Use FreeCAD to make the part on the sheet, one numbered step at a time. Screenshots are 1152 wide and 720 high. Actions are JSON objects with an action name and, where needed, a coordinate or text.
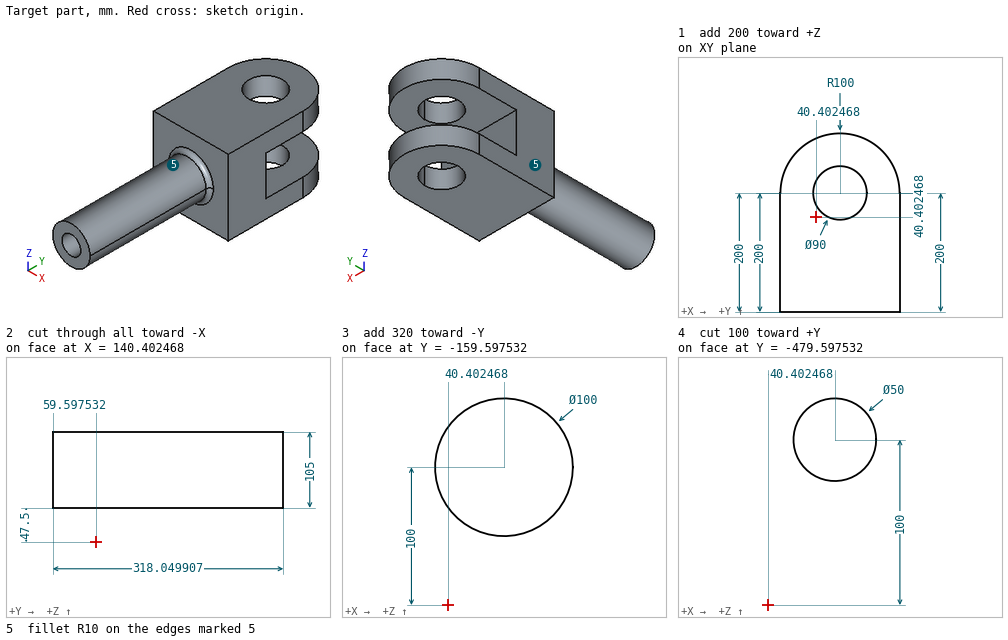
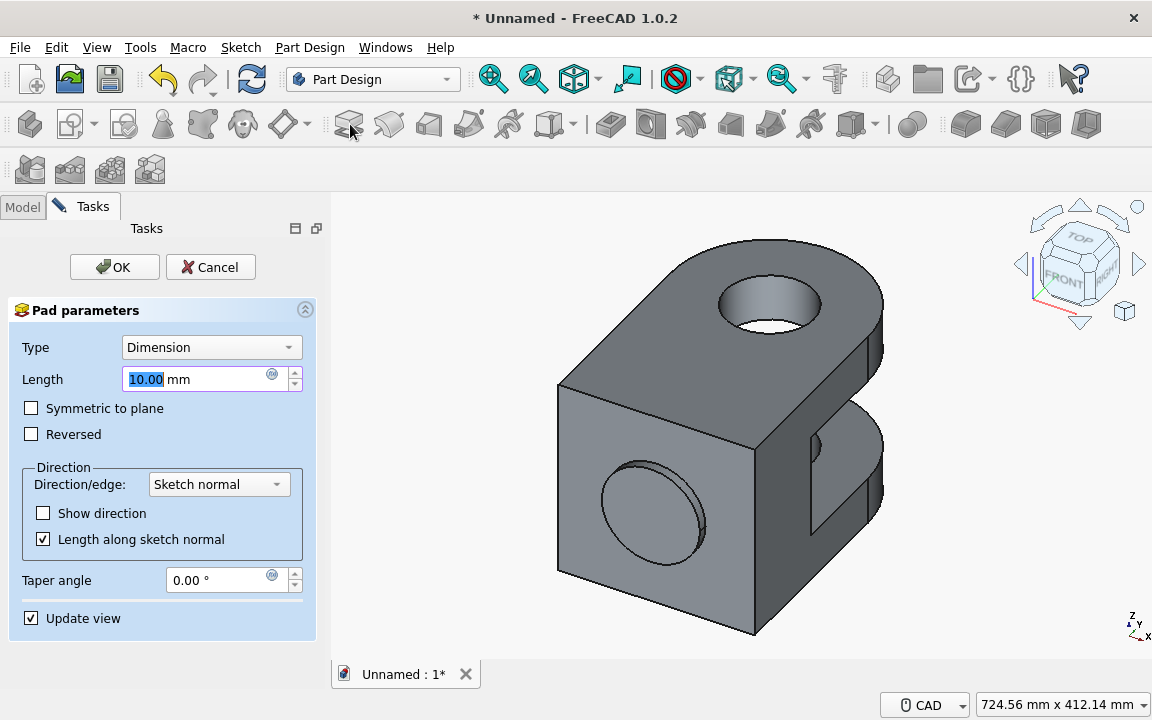
{"action": "type", "text": "320"}
{"action": "key", "text": "Tab"}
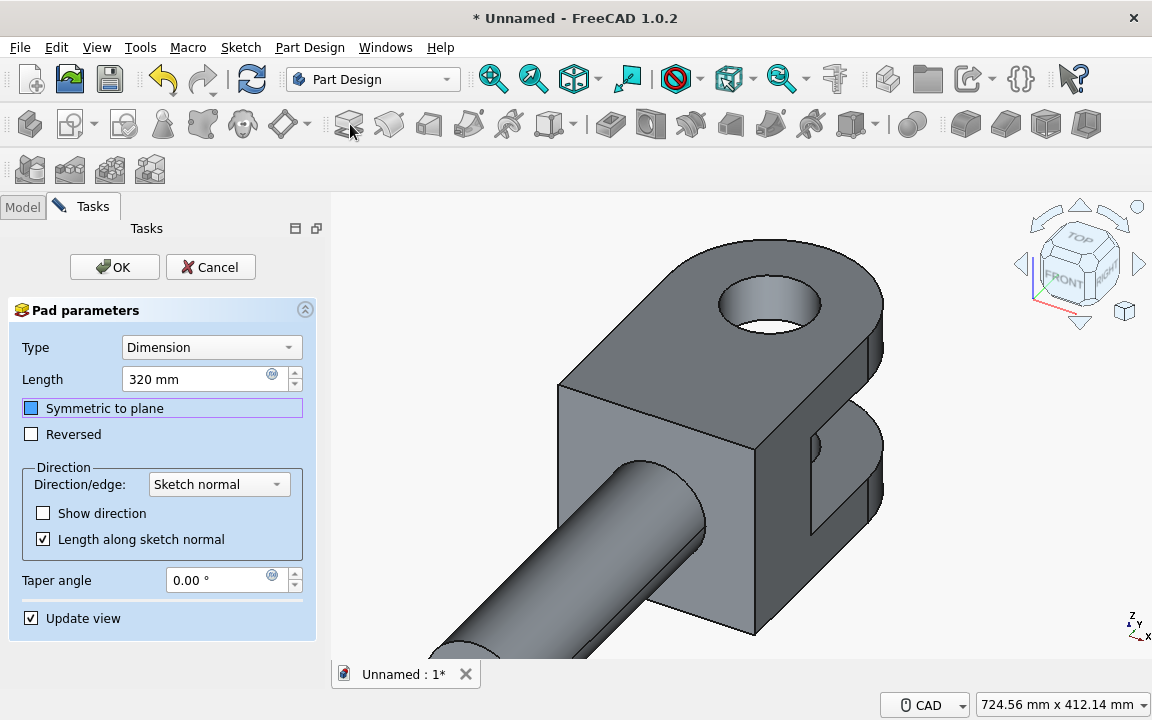
{"action": "left_click", "coordinate": [115, 267]}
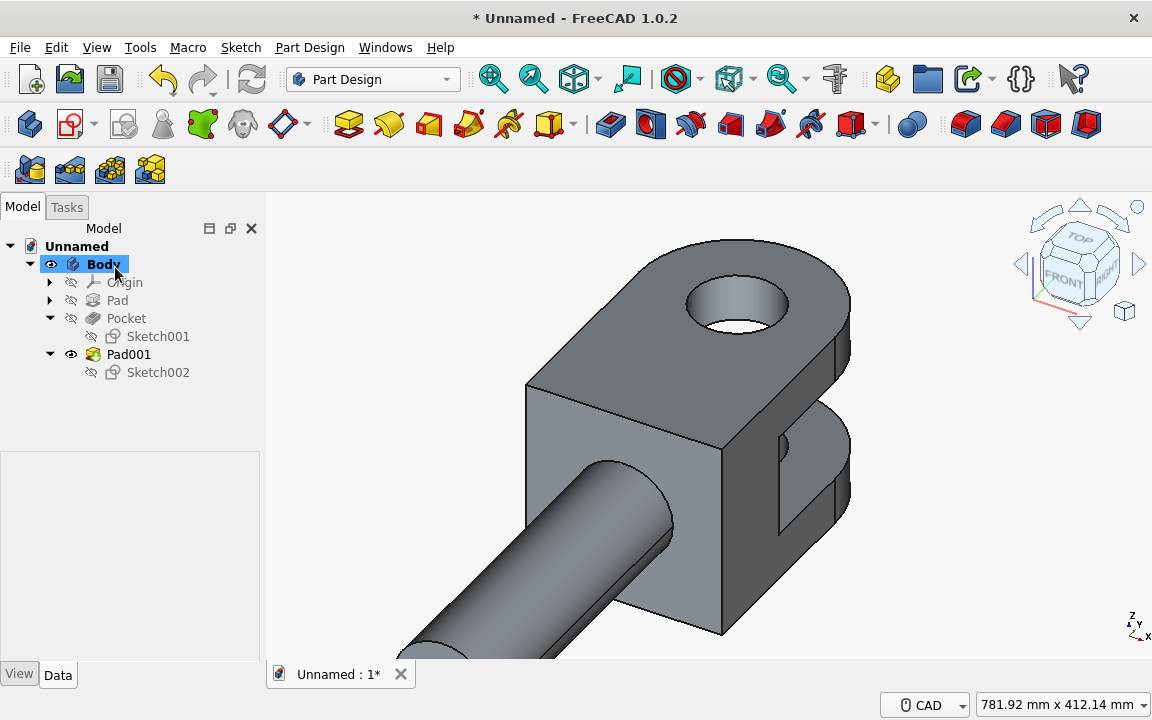
{"action": "key", "text": "v f"}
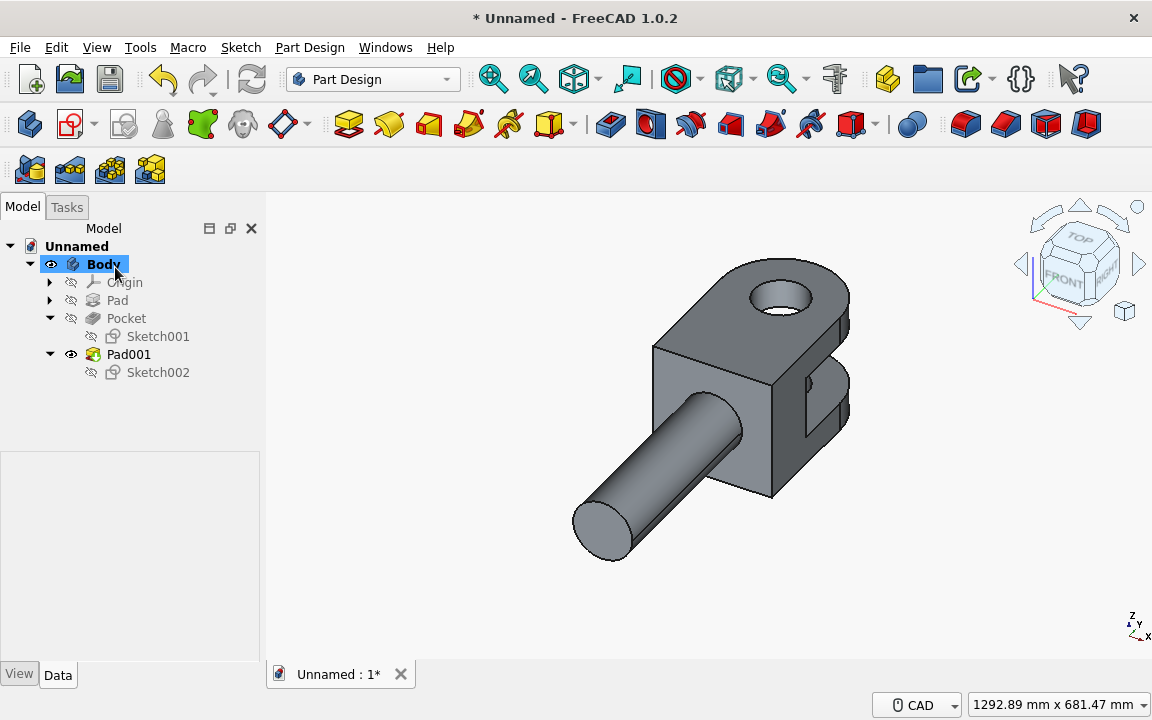
{"action": "left_click", "coordinate": [603, 530]}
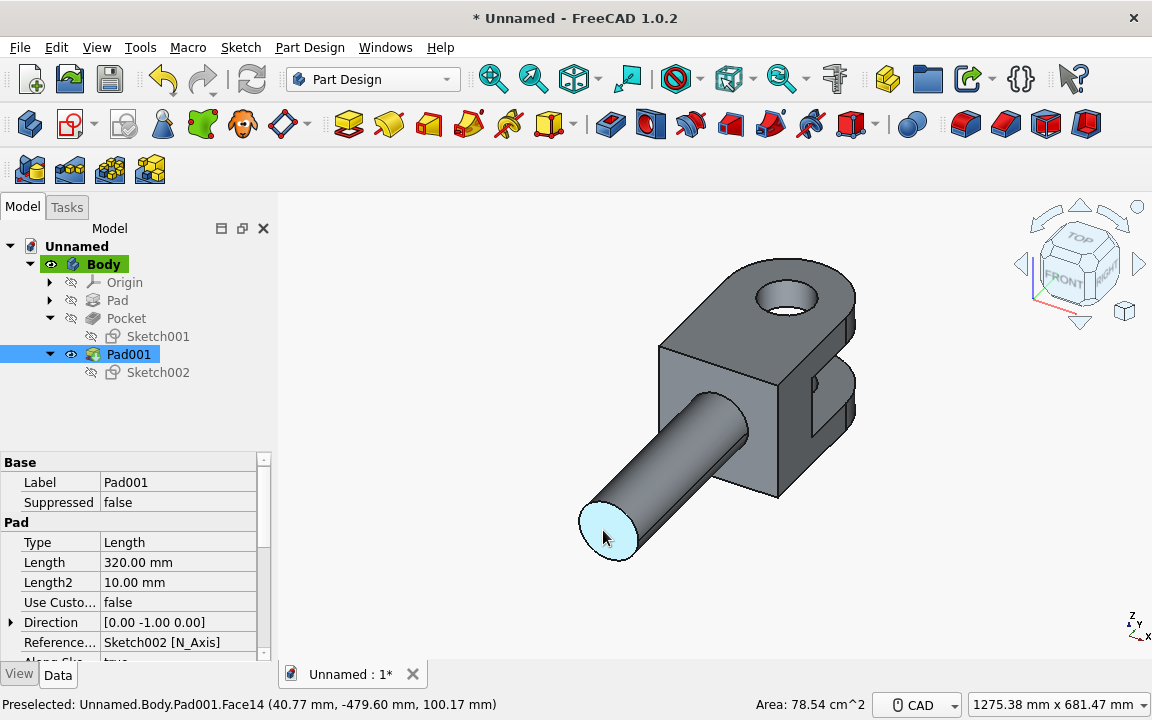
{"action": "left_click", "coordinate": [70, 124]}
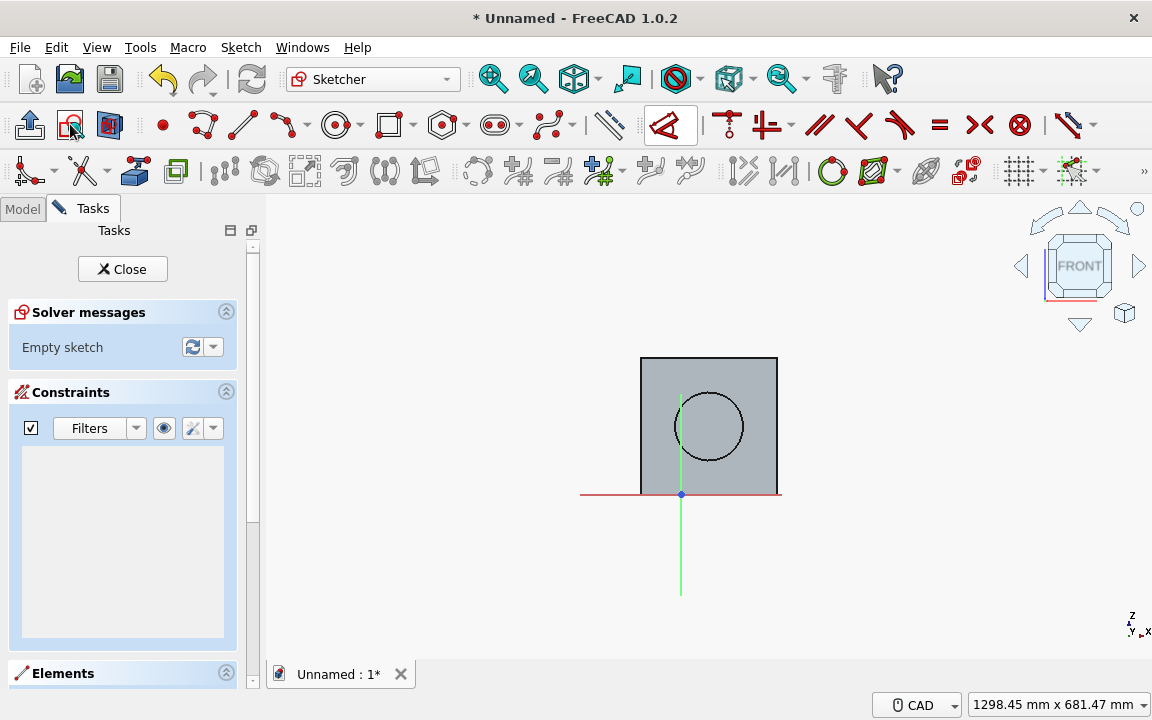
{"action": "scroll", "coordinate": [718, 427], "scroll_direction": "up", "scroll_amount": 11}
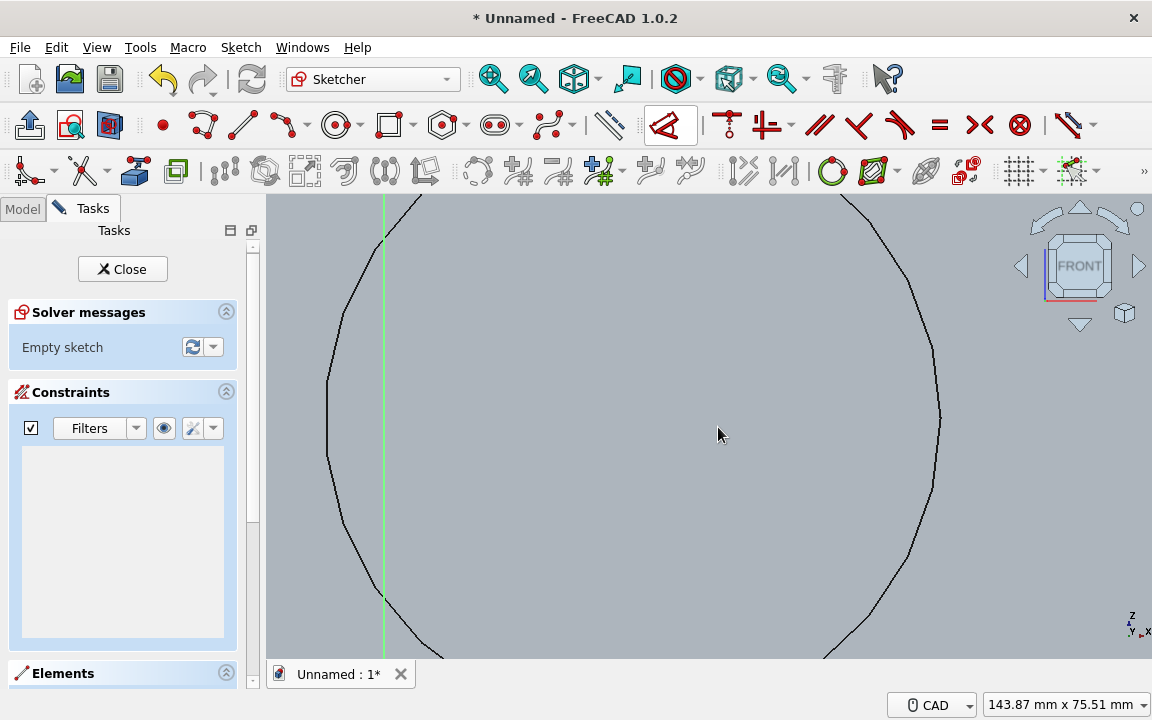
{"action": "key", "text": "g c"}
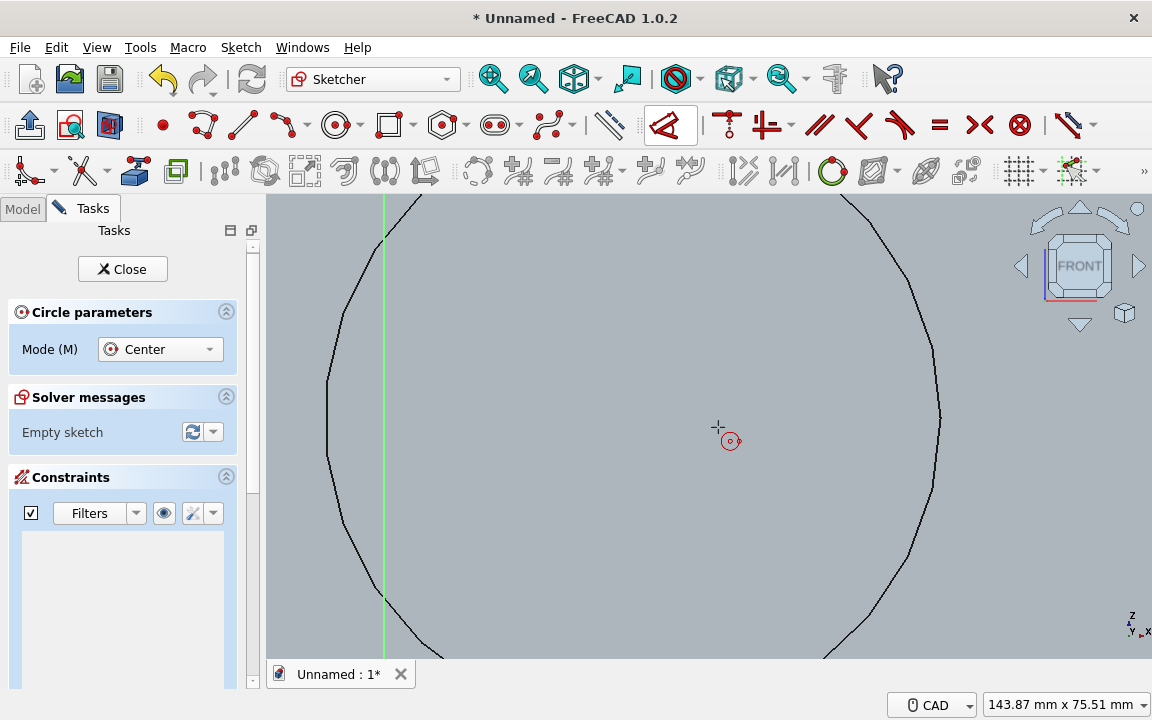
{"action": "left_click", "coordinate": [633, 418]}
{"action": "mouse_move", "coordinate": [742, 310]}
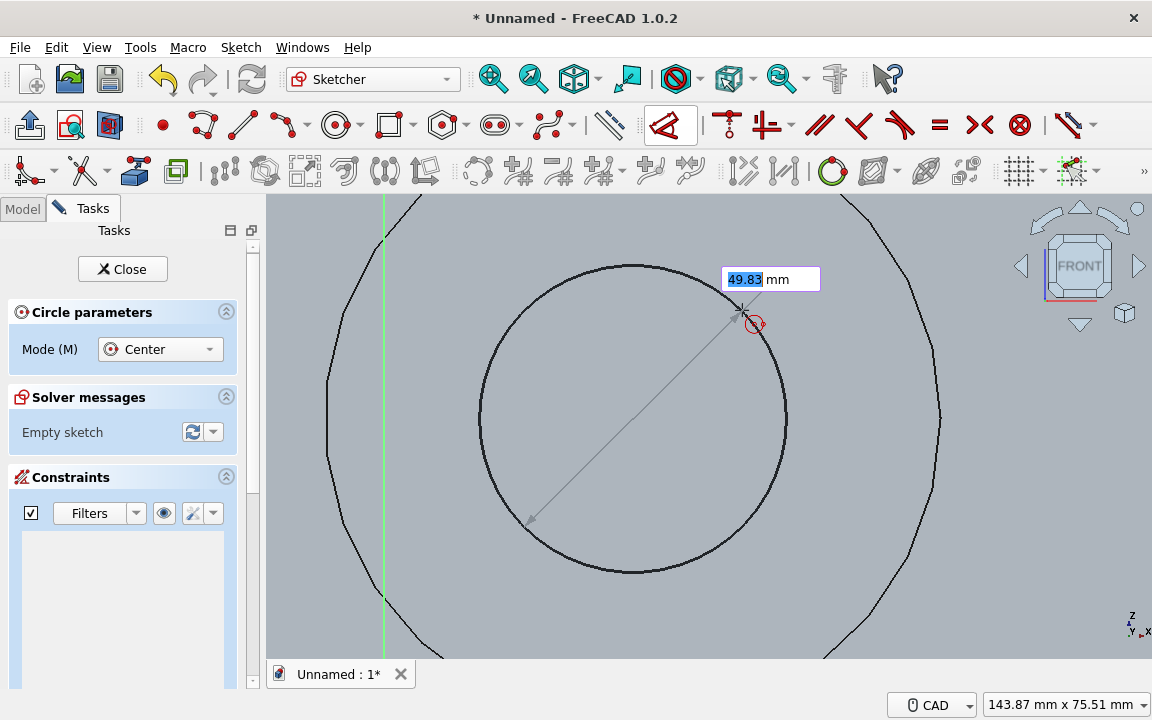
{"action": "type", "text": "50"}
{"action": "key", "text": "Return"}
{"action": "key", "text": "Escape"}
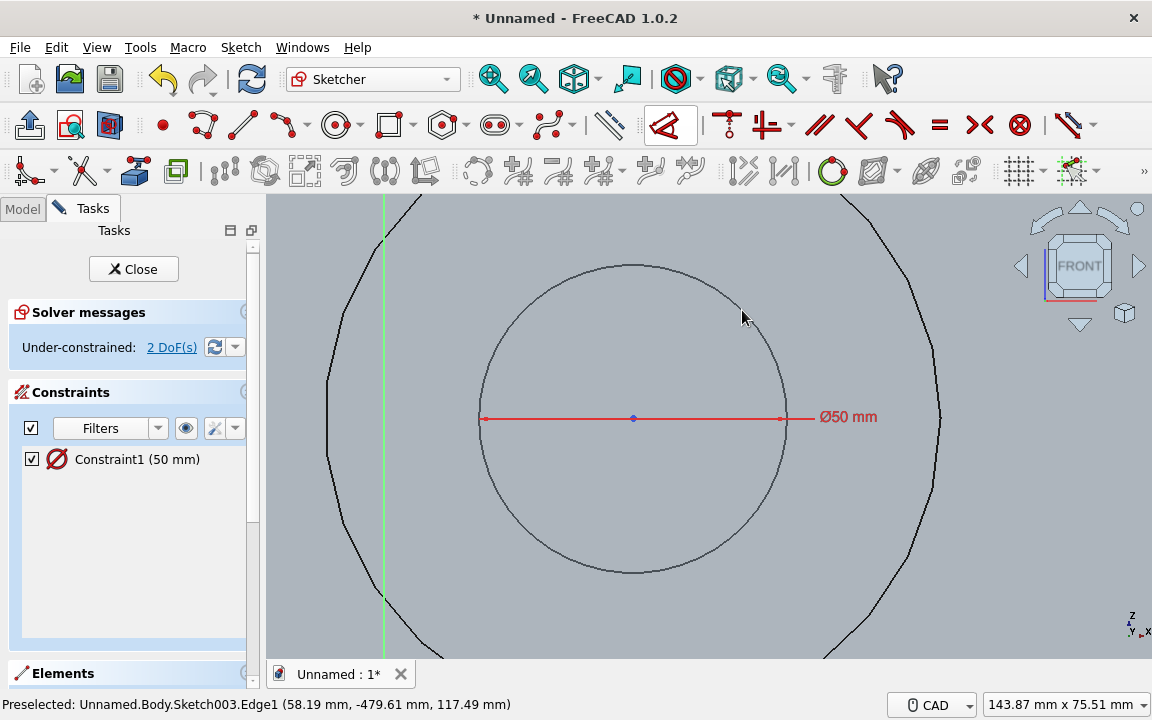
{"action": "left_click", "coordinate": [633, 419]}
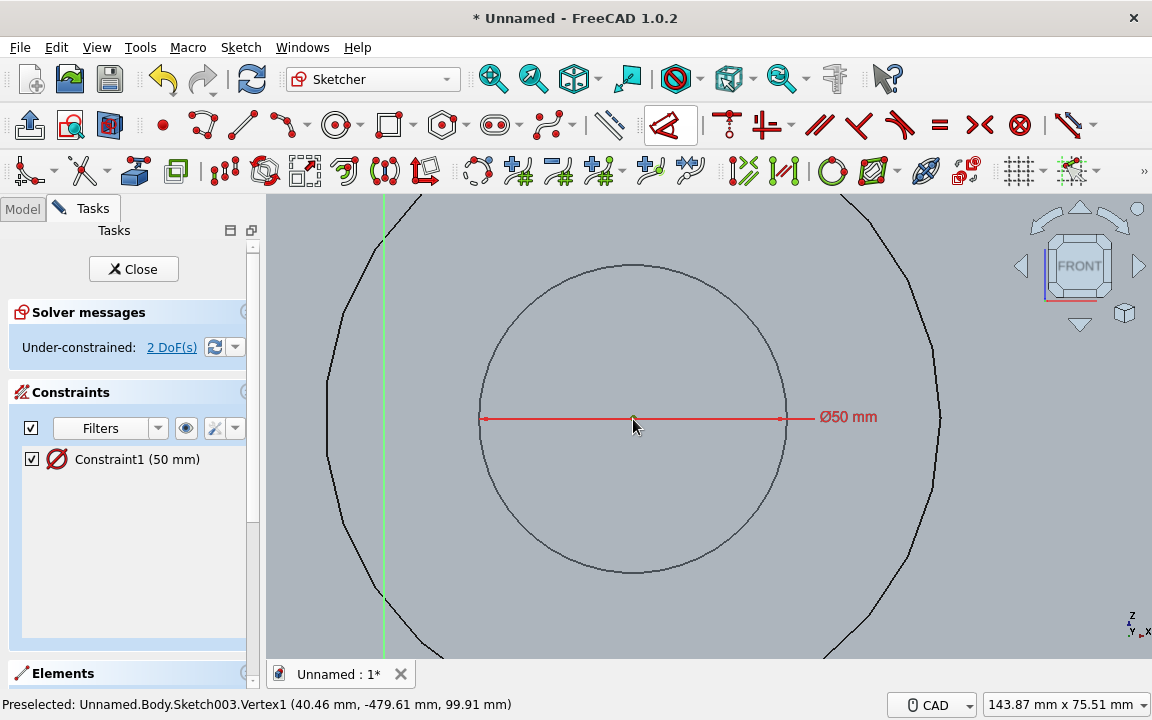
{"action": "key", "text": "i"}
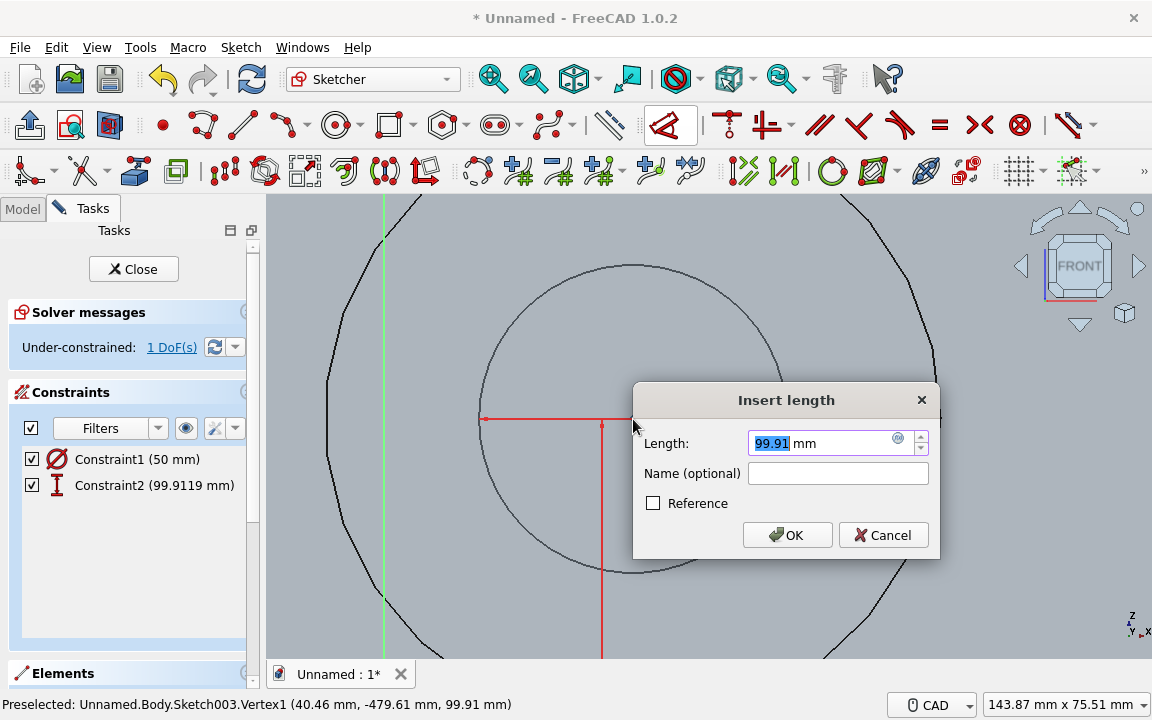
{"action": "type", "text": "100"}
{"action": "key", "text": "Return"}